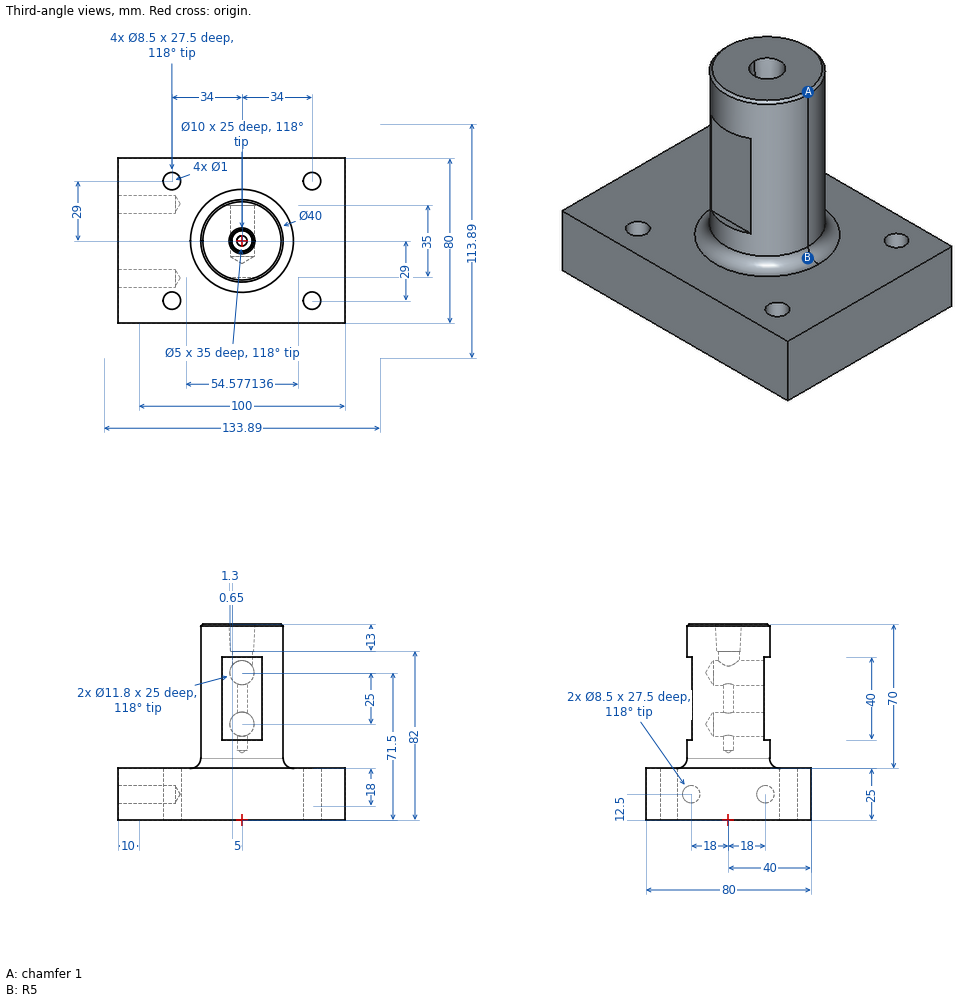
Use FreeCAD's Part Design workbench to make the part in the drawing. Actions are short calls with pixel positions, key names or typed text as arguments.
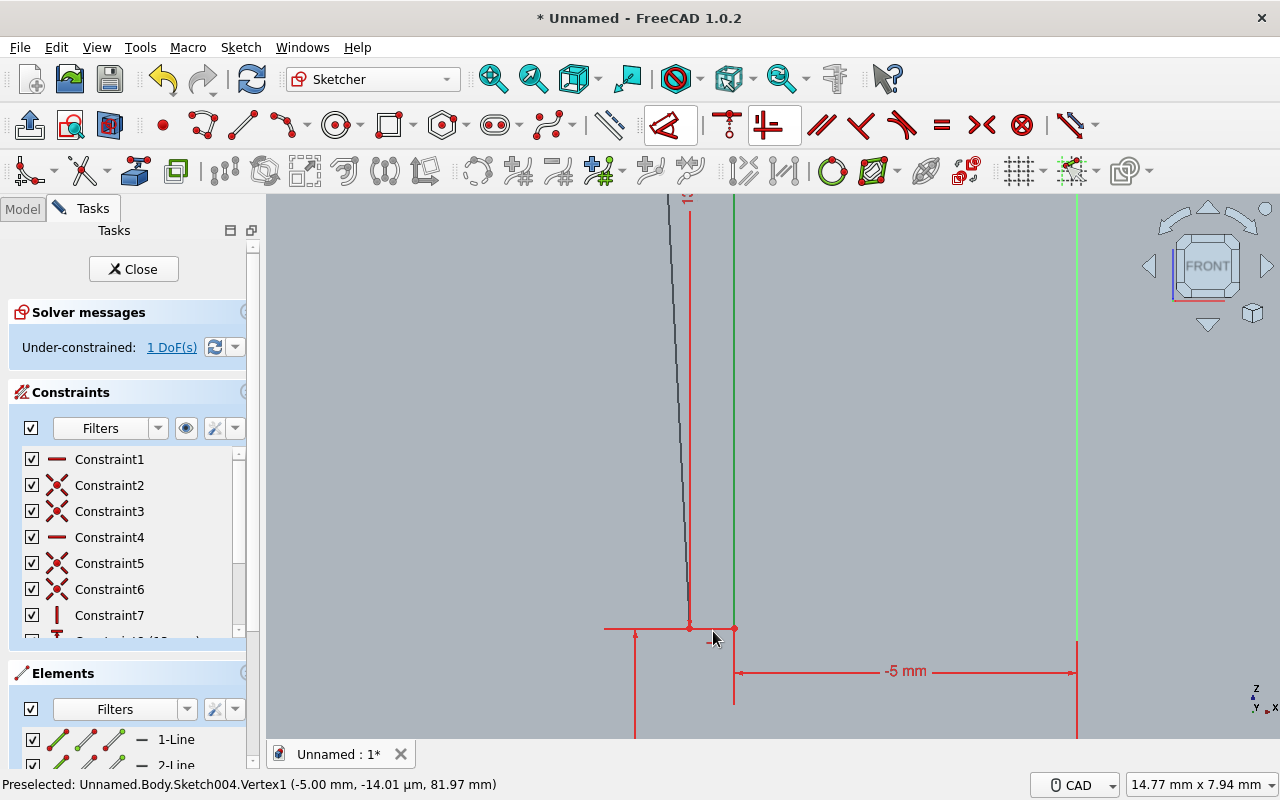
click(712, 629)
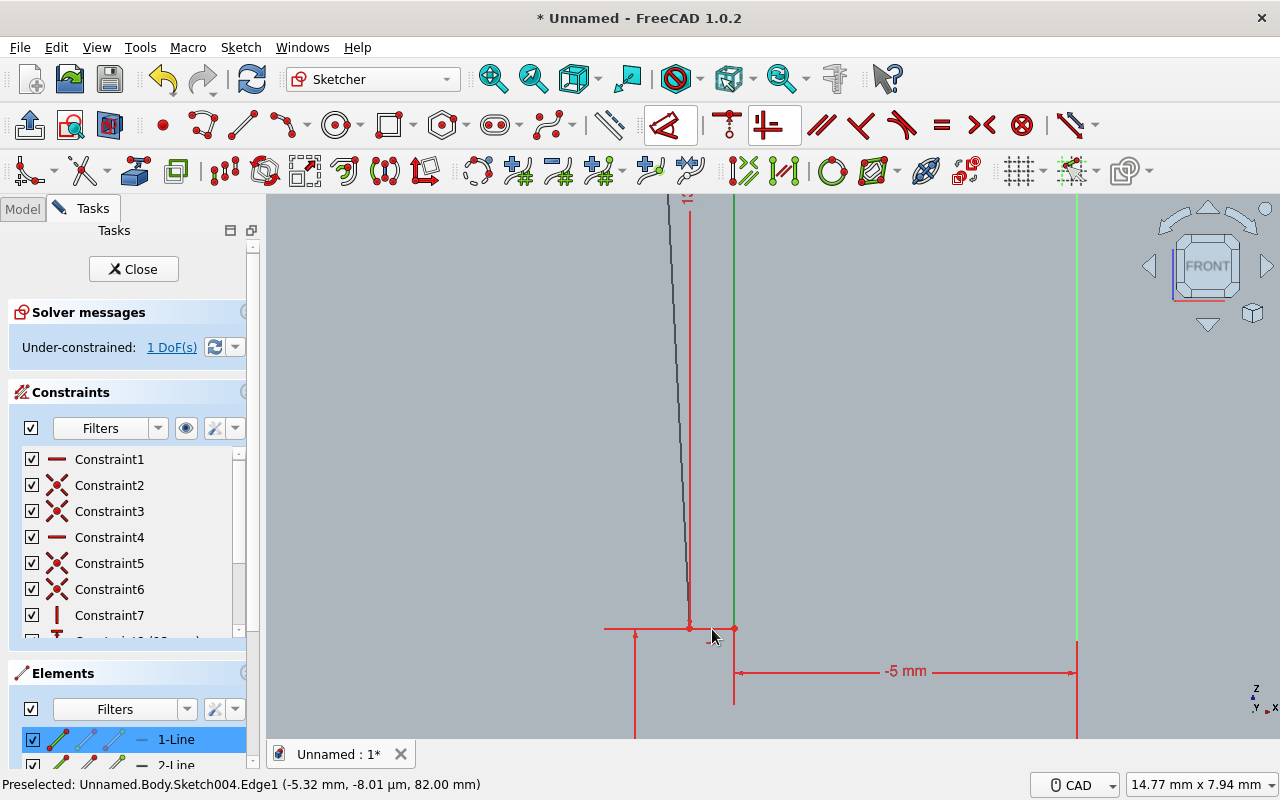
key(l)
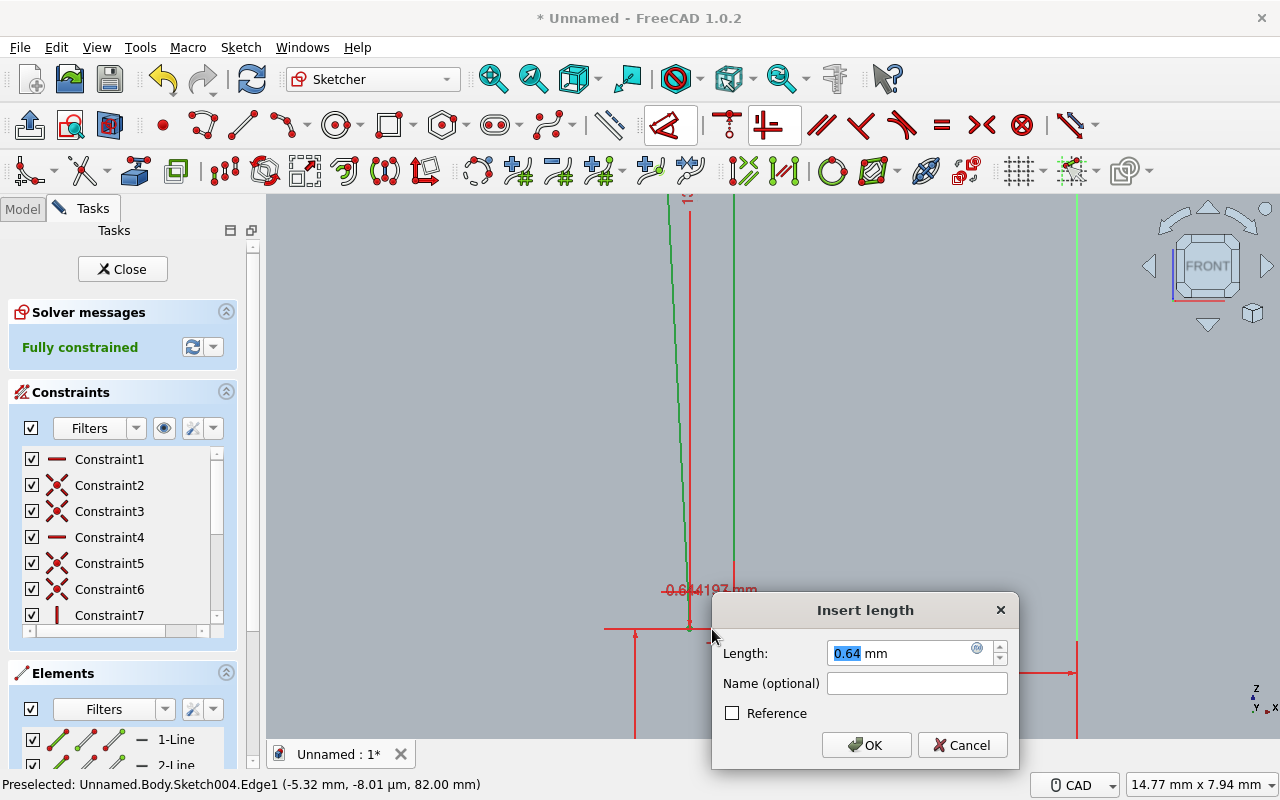
text(0.65)
key(Return)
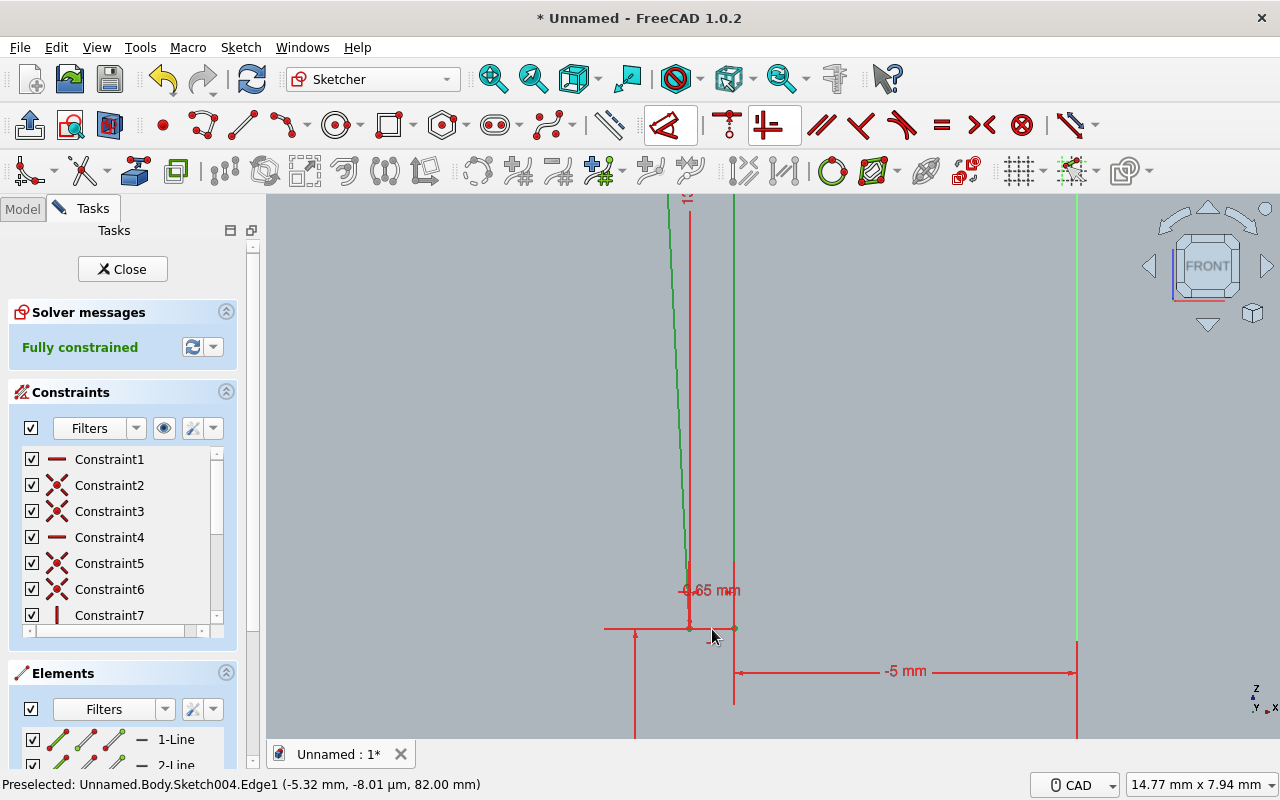
click(123, 269)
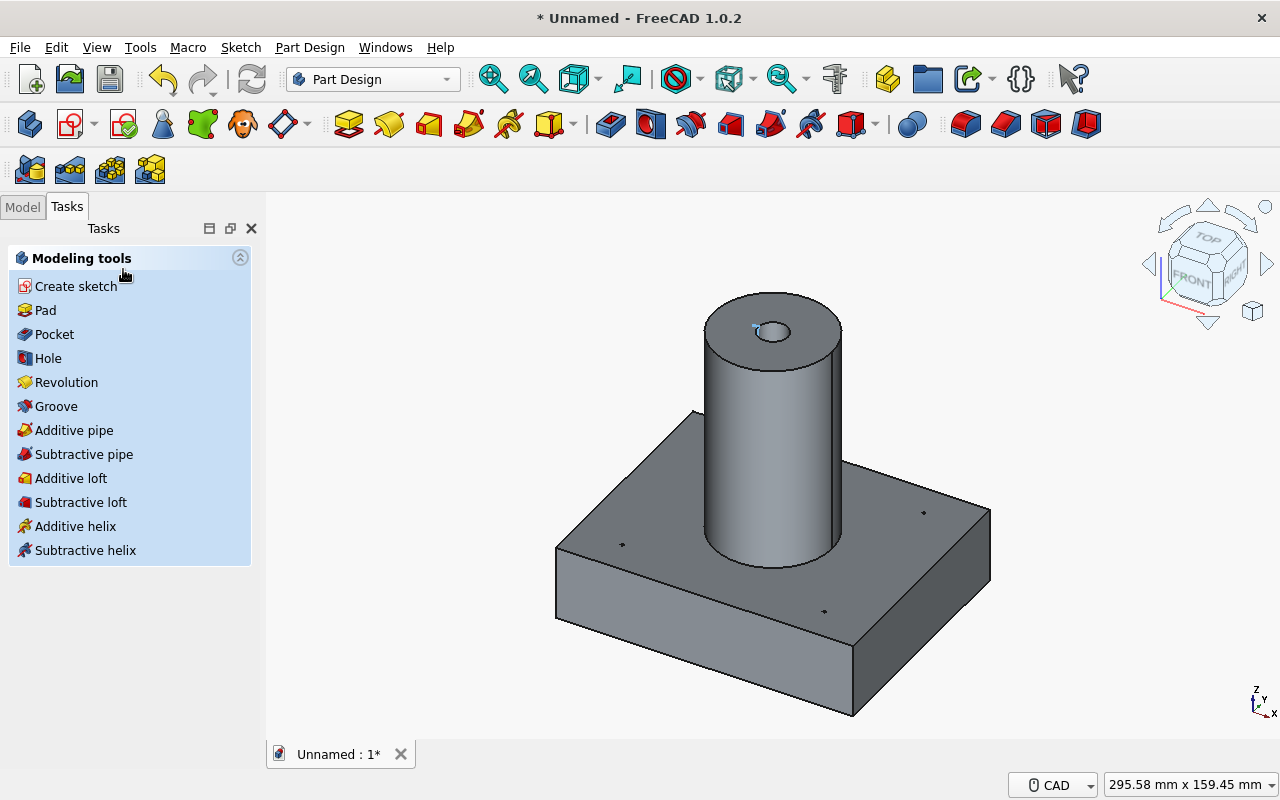
click(692, 124)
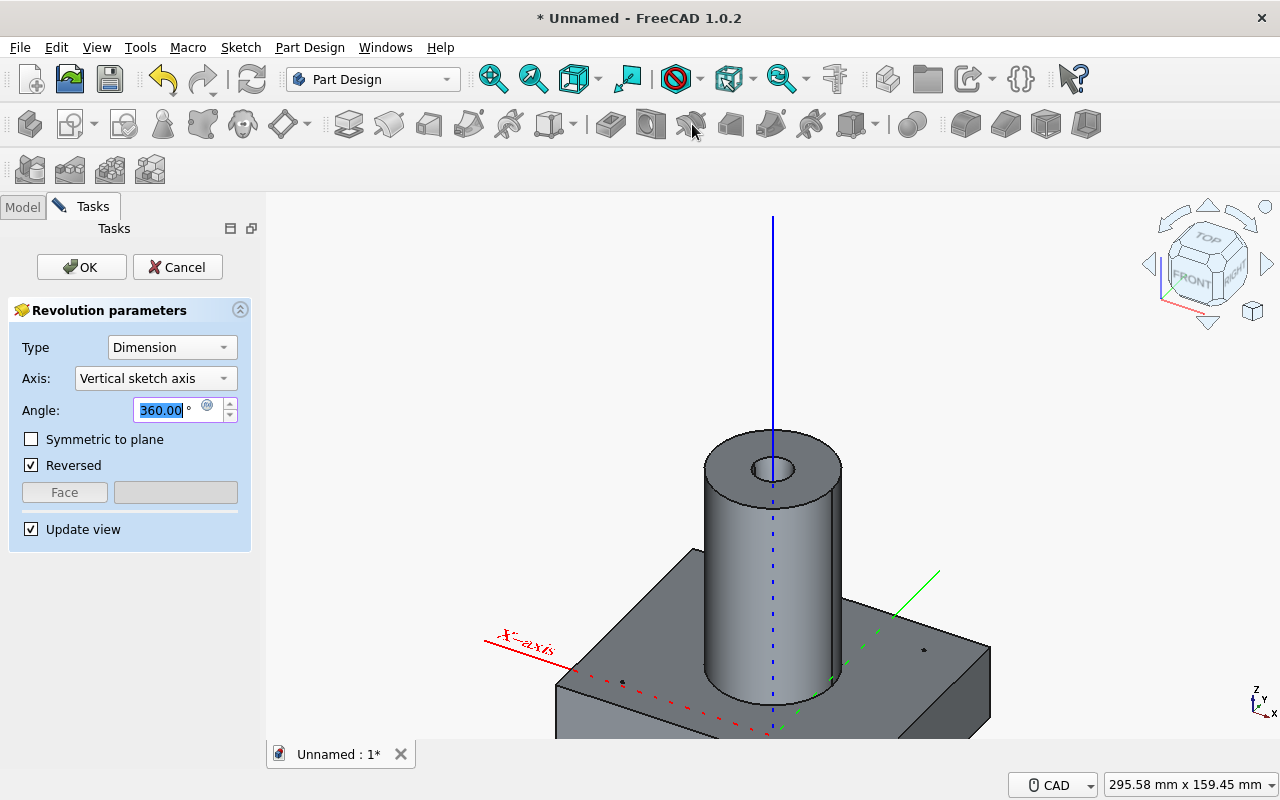
click(82, 267)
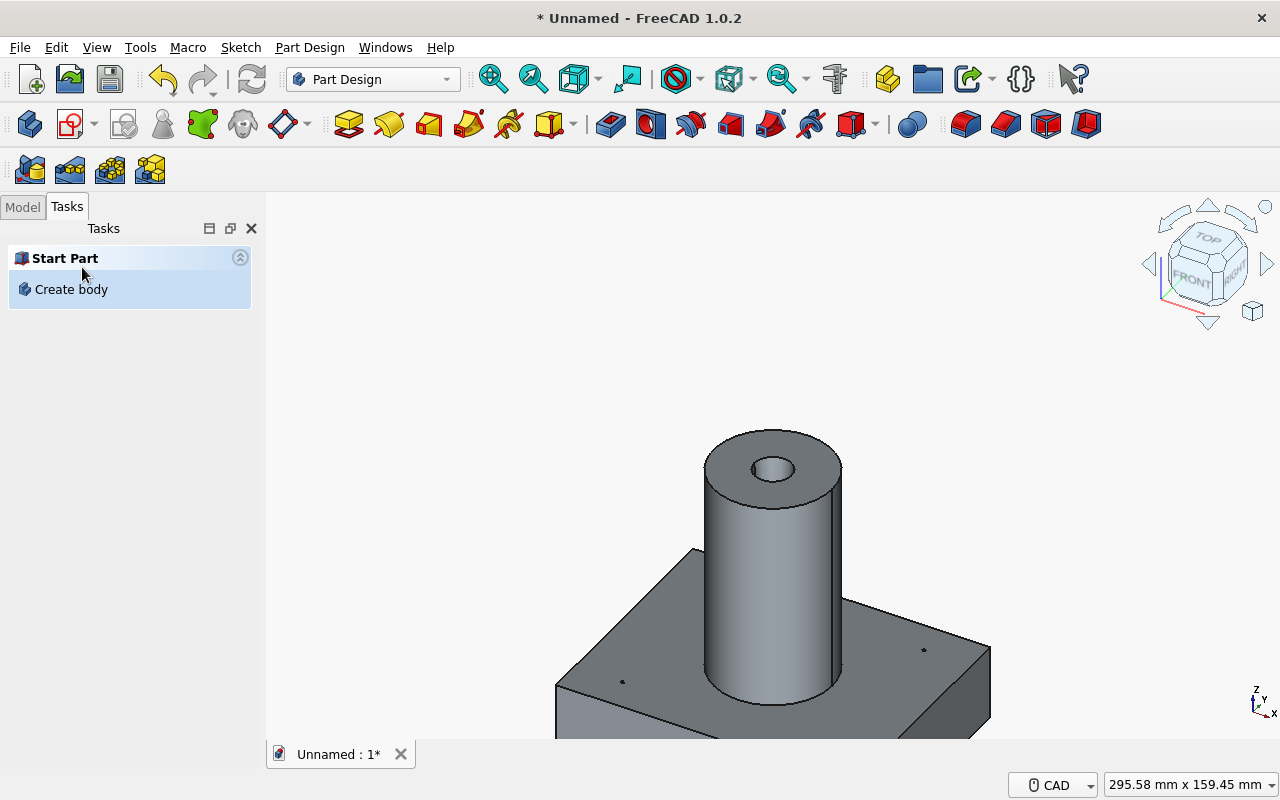
click(494, 80)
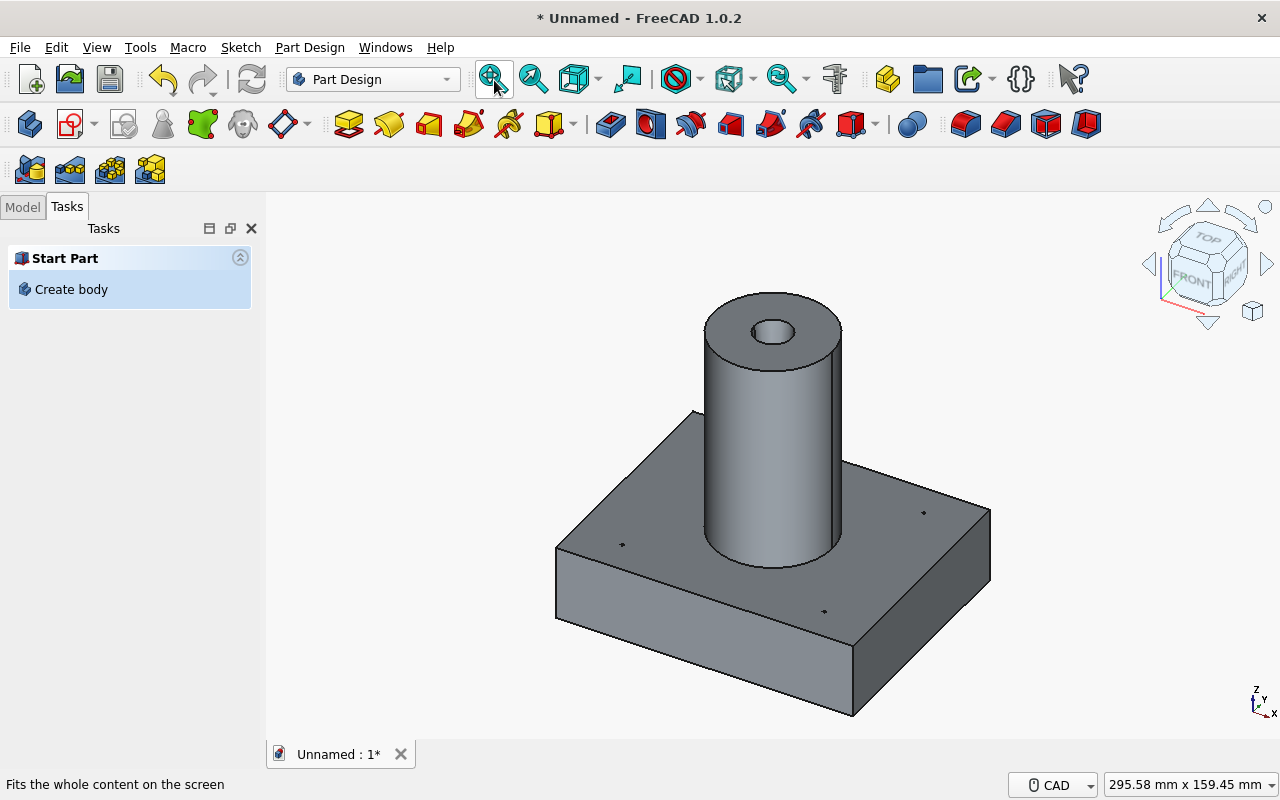
click(23, 206)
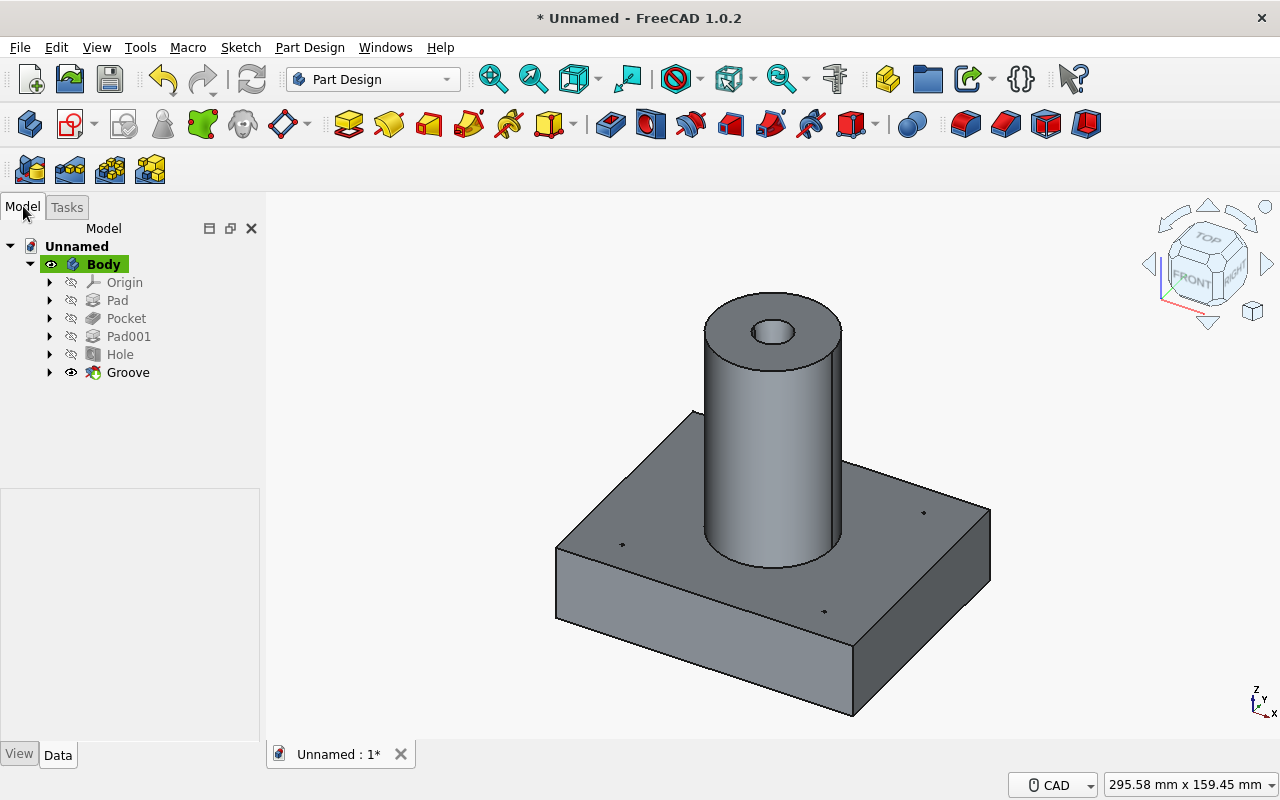
click(50, 282)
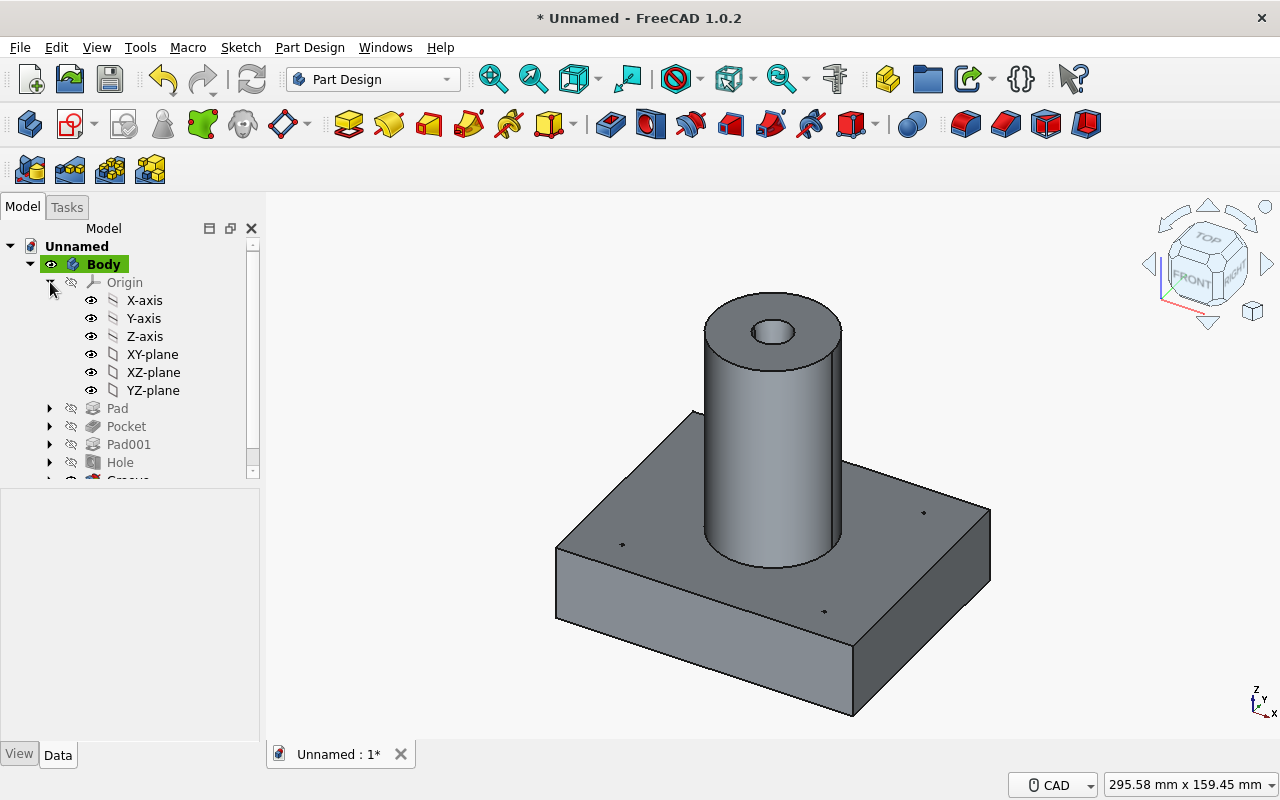
click(136, 354)